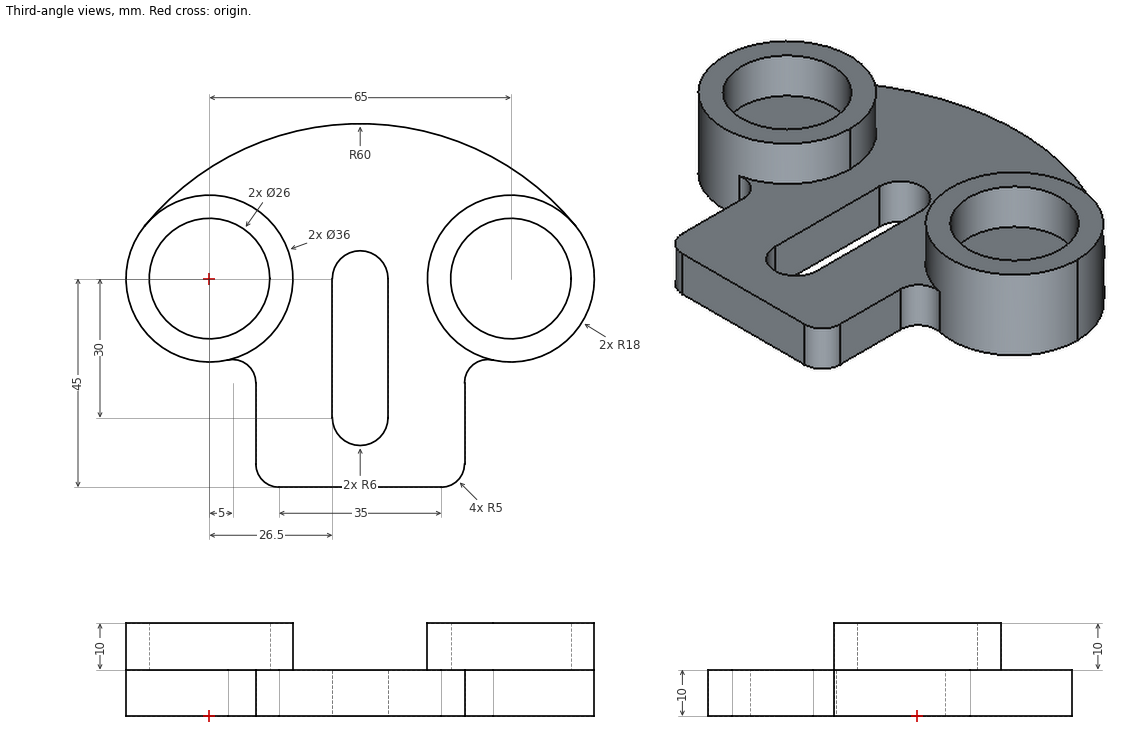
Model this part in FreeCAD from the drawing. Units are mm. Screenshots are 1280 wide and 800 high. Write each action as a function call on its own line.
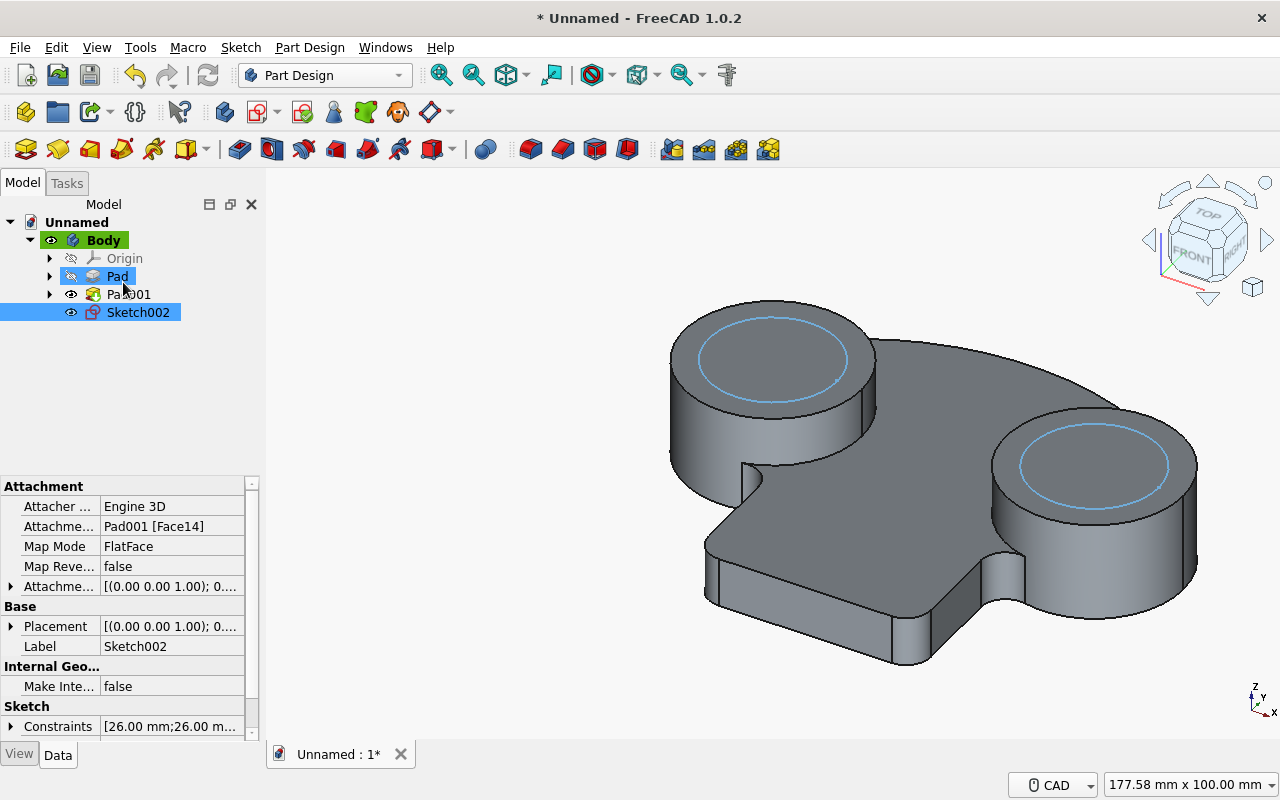
click(240, 150)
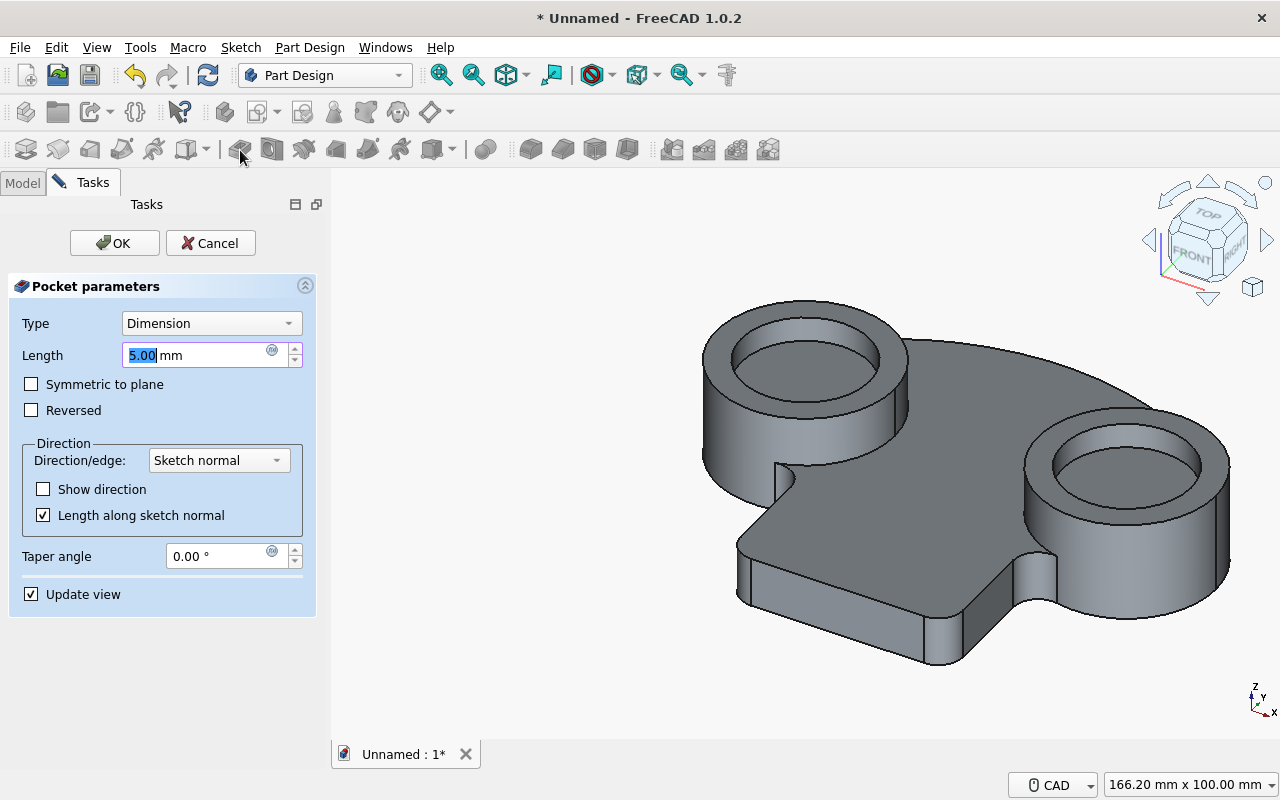
text(10)
key(Tab)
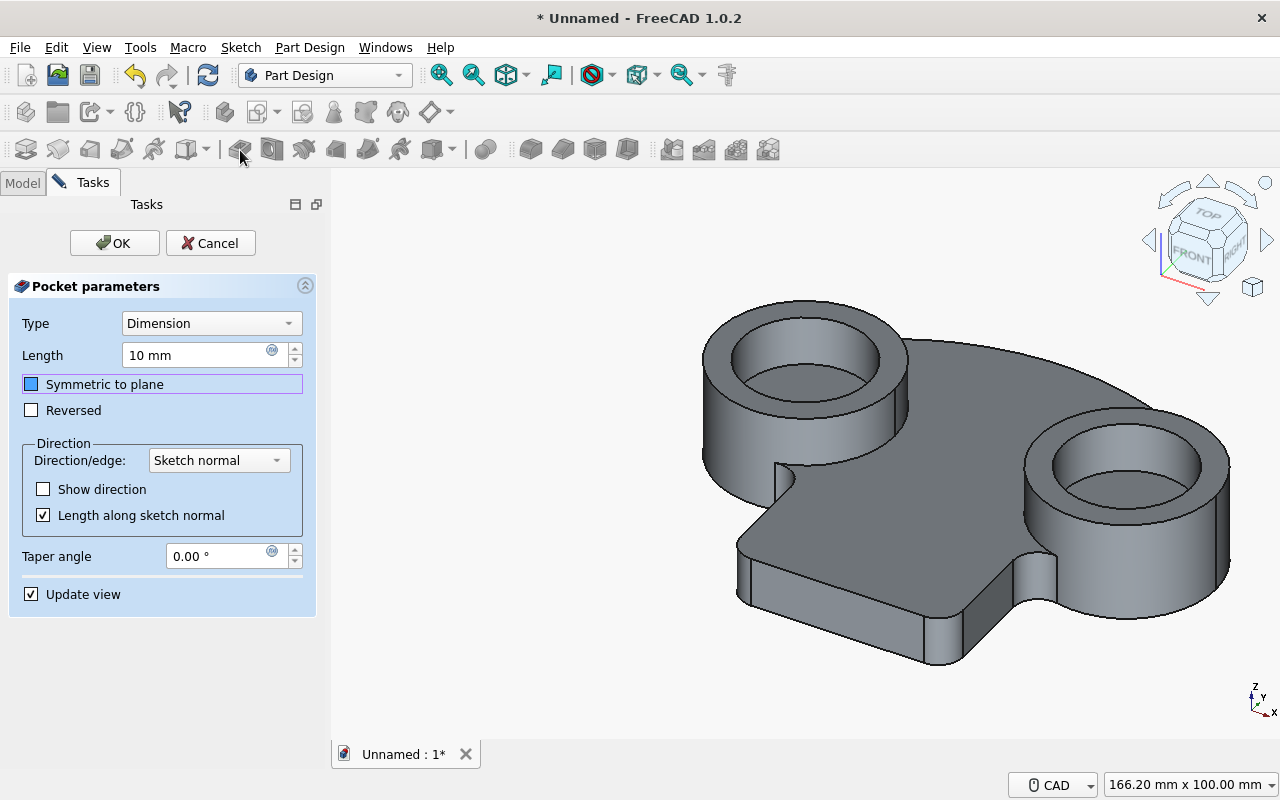
click(115, 243)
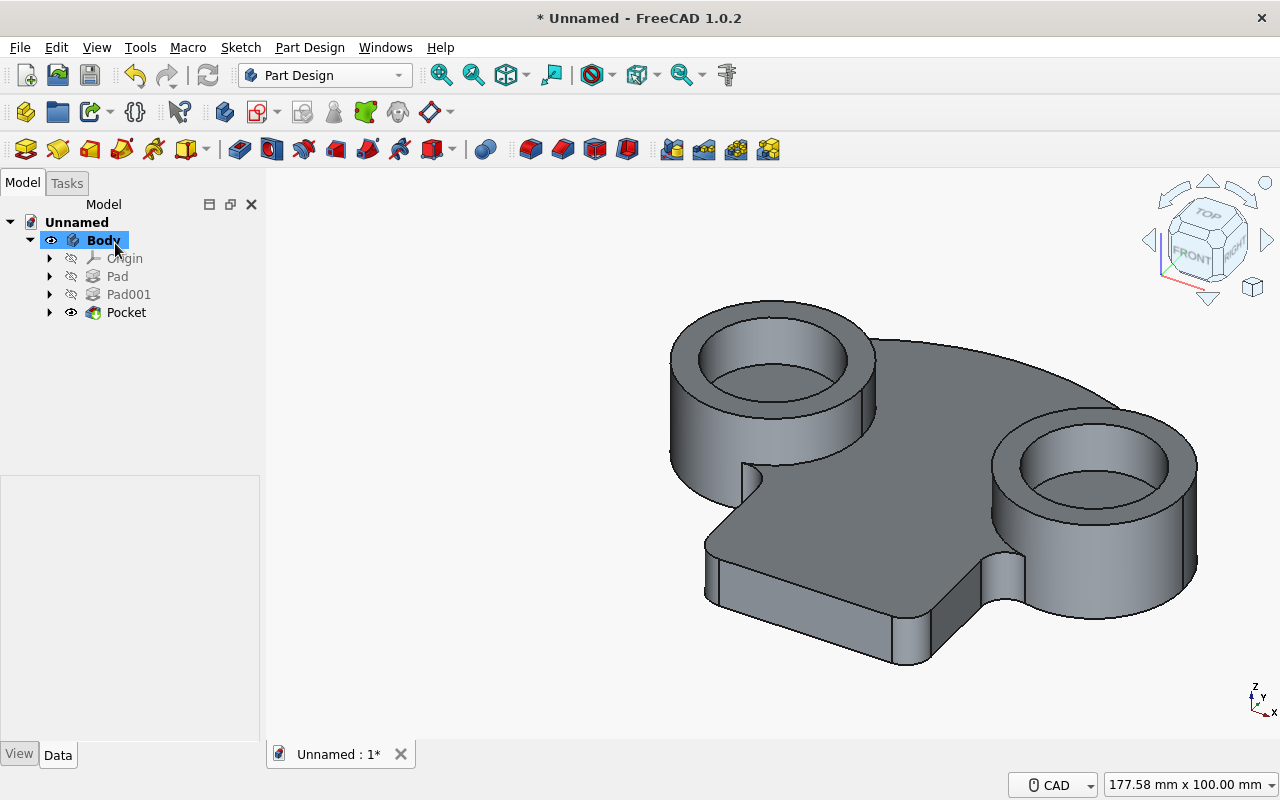
click(885, 507)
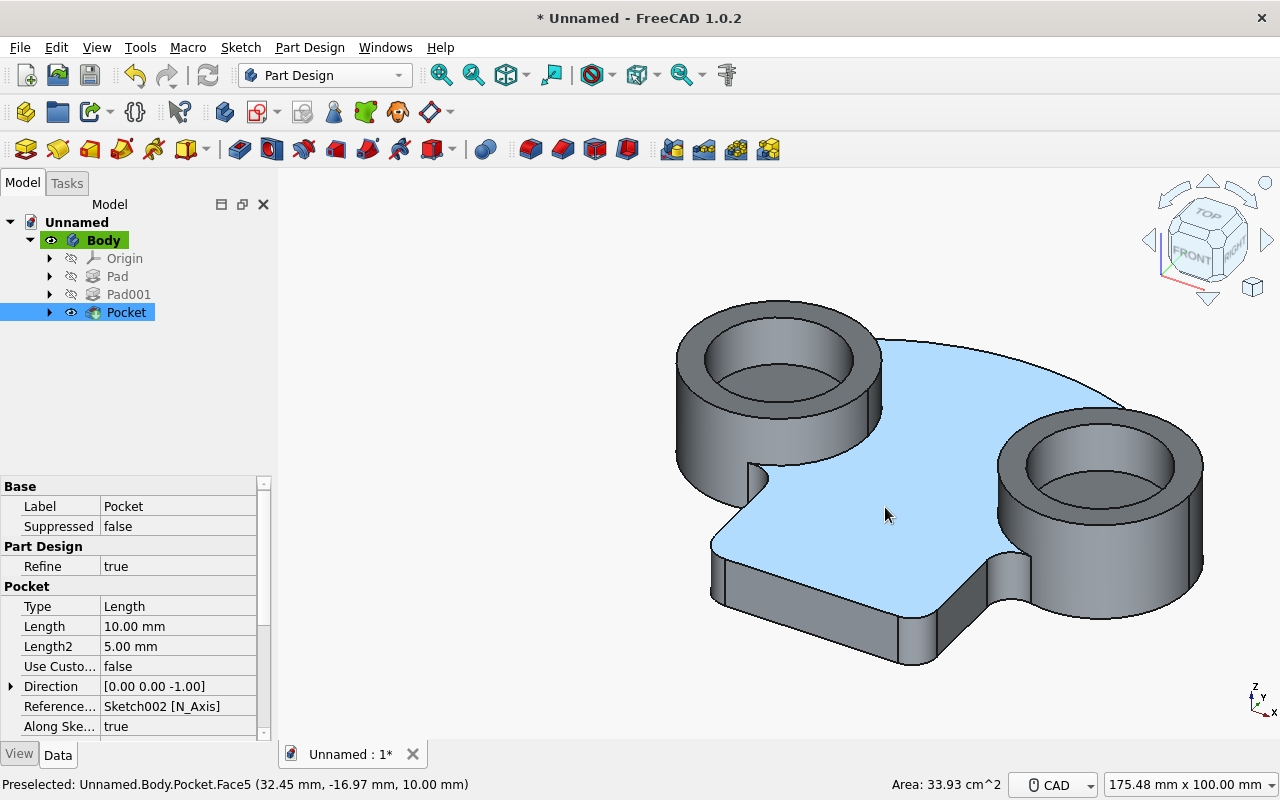
click(258, 112)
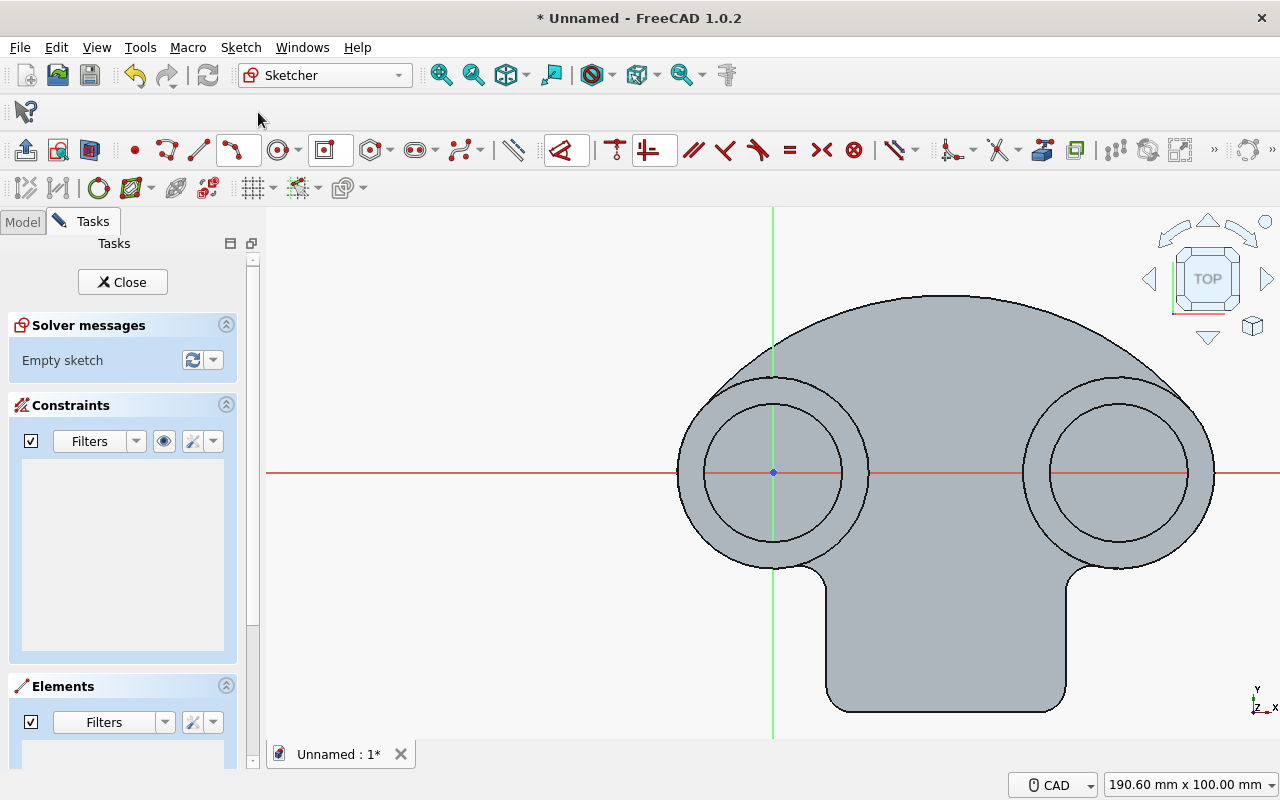
scroll(1115, 711, up, 2)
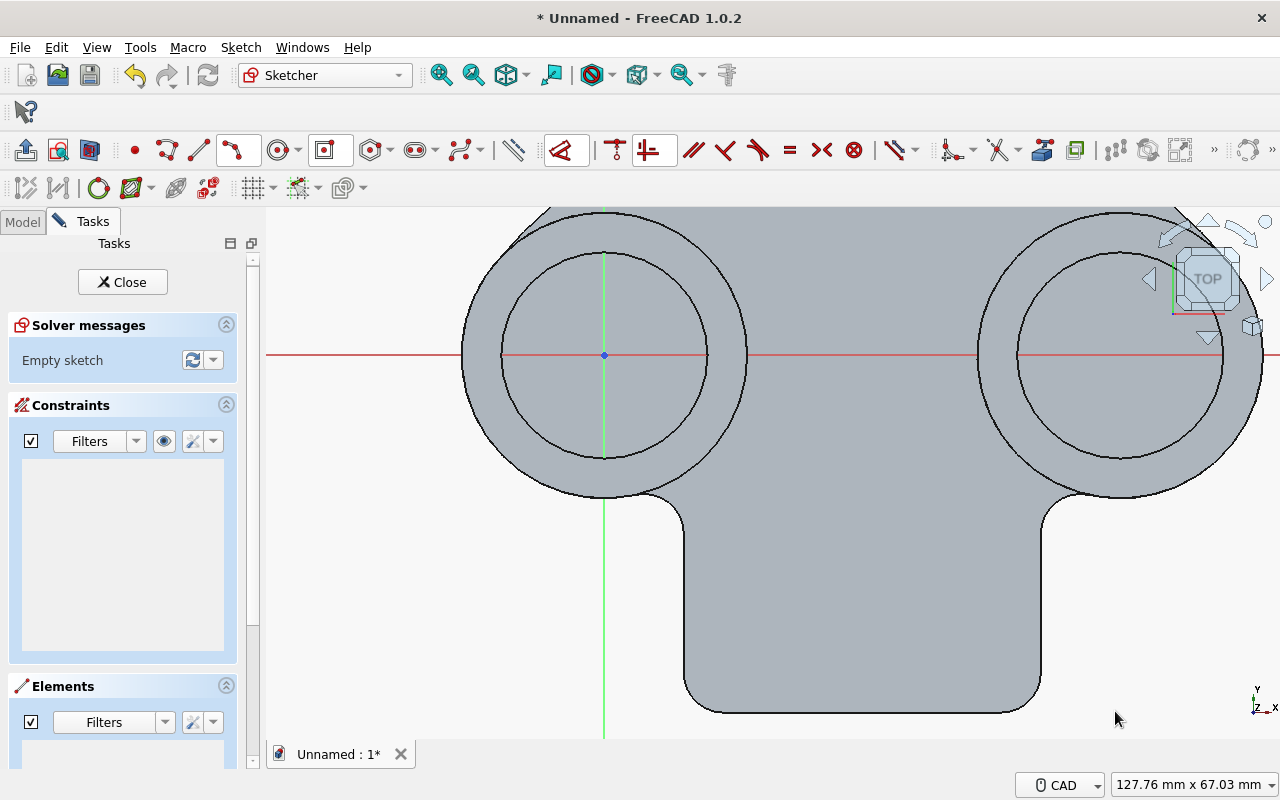
click(416, 150)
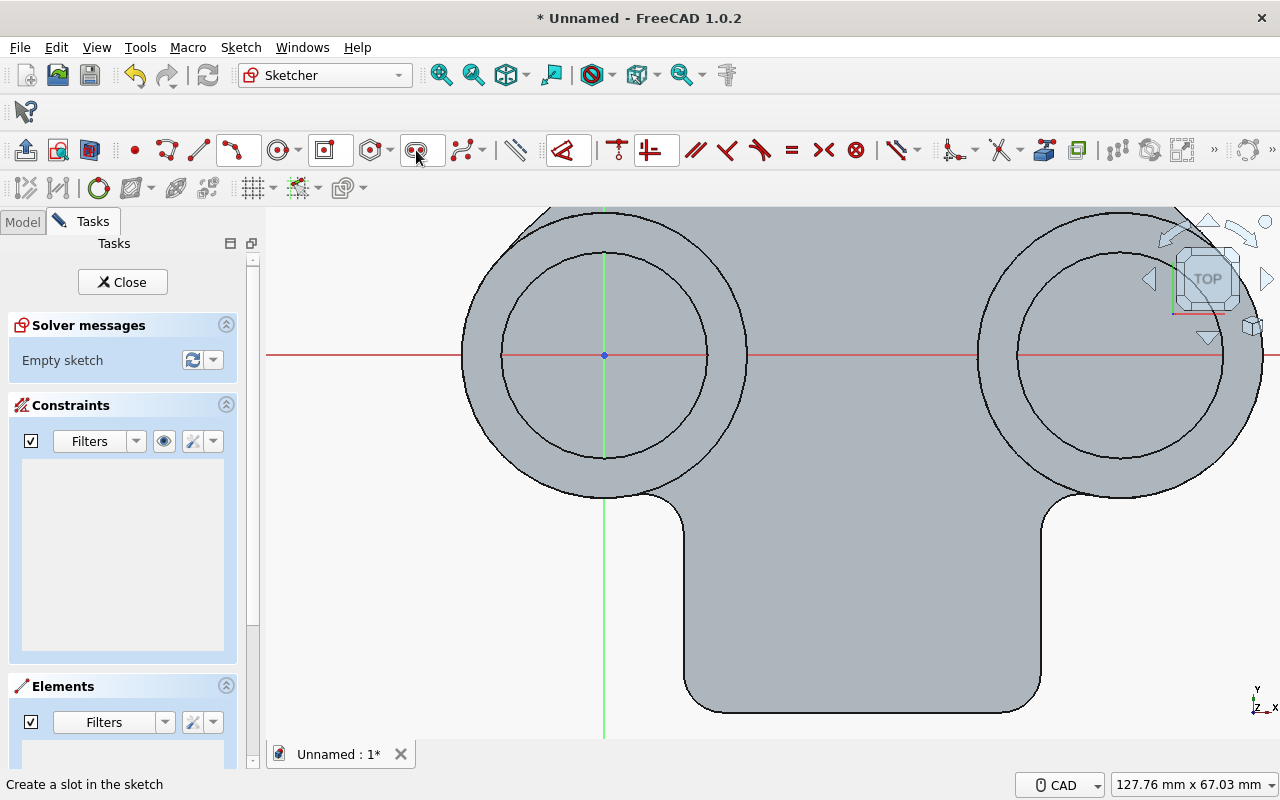
click(862, 594)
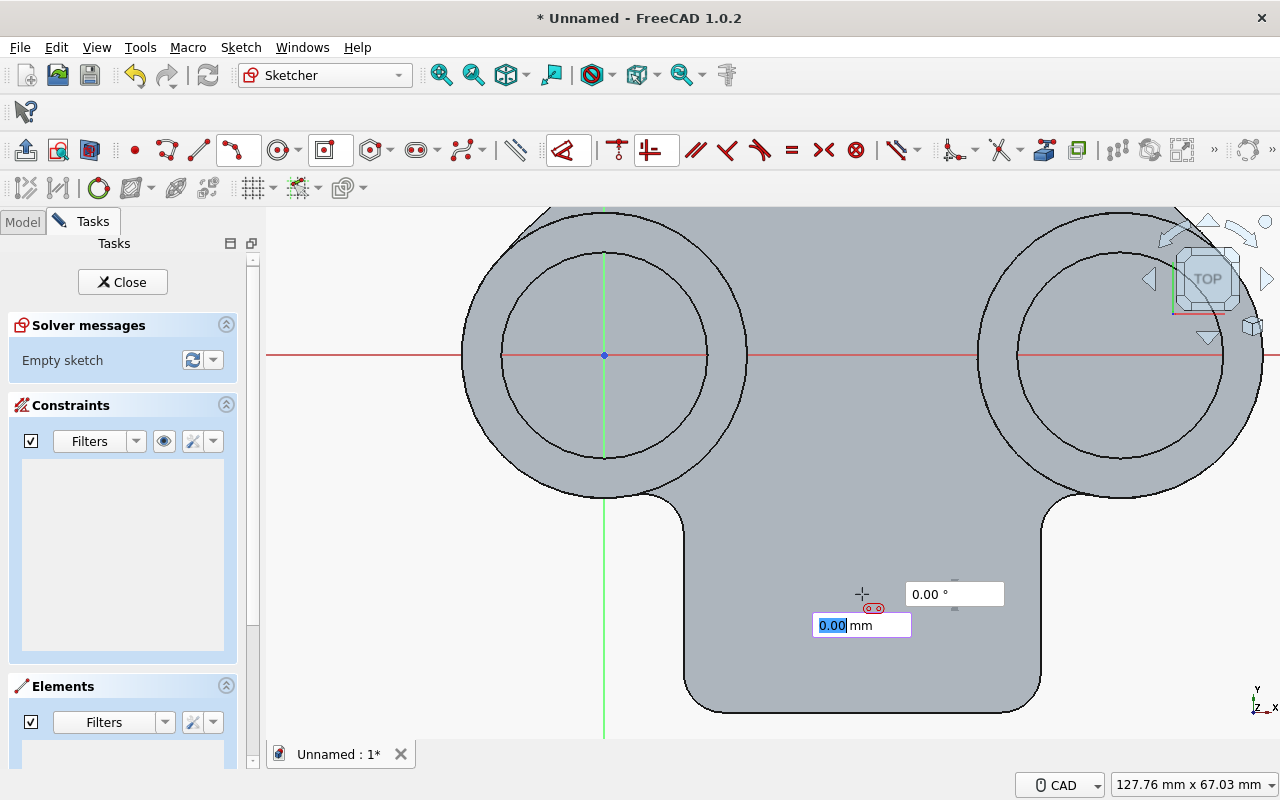
click(862, 355)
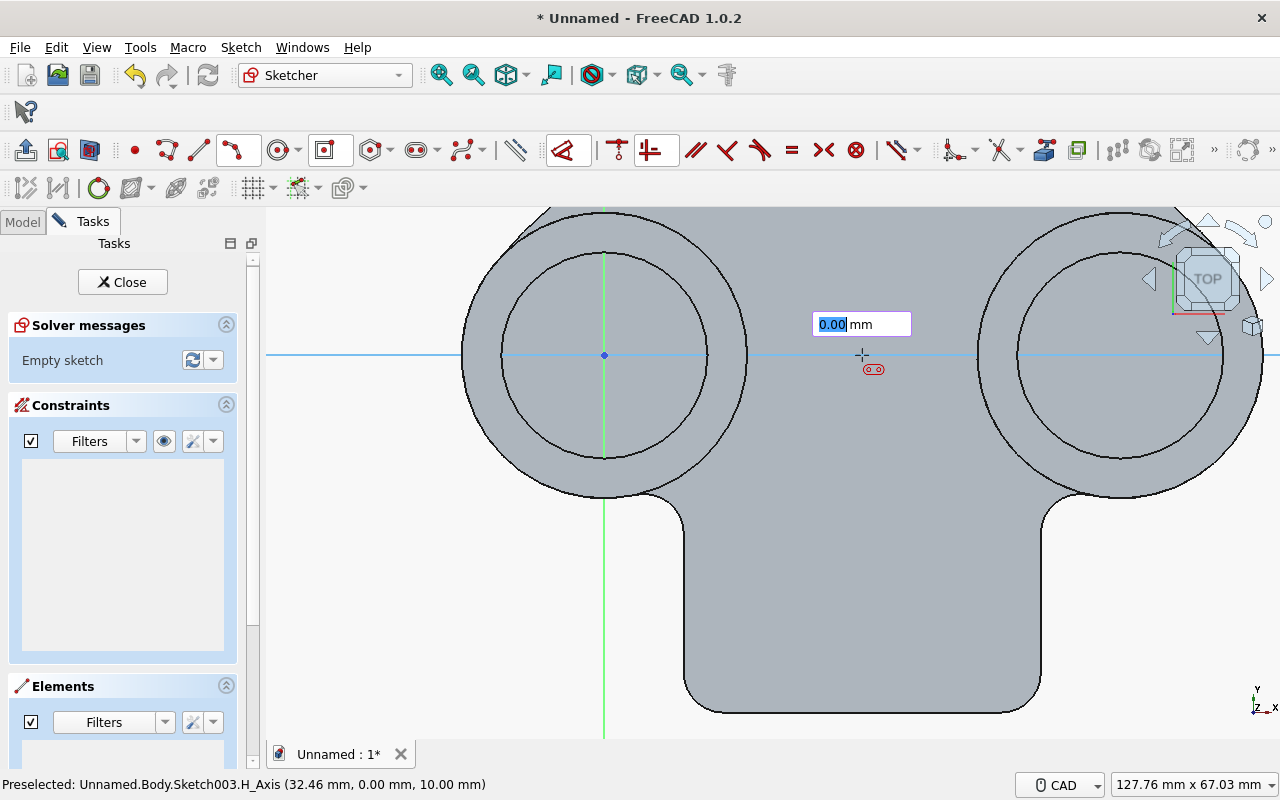
click(815, 475)
key(Escape)